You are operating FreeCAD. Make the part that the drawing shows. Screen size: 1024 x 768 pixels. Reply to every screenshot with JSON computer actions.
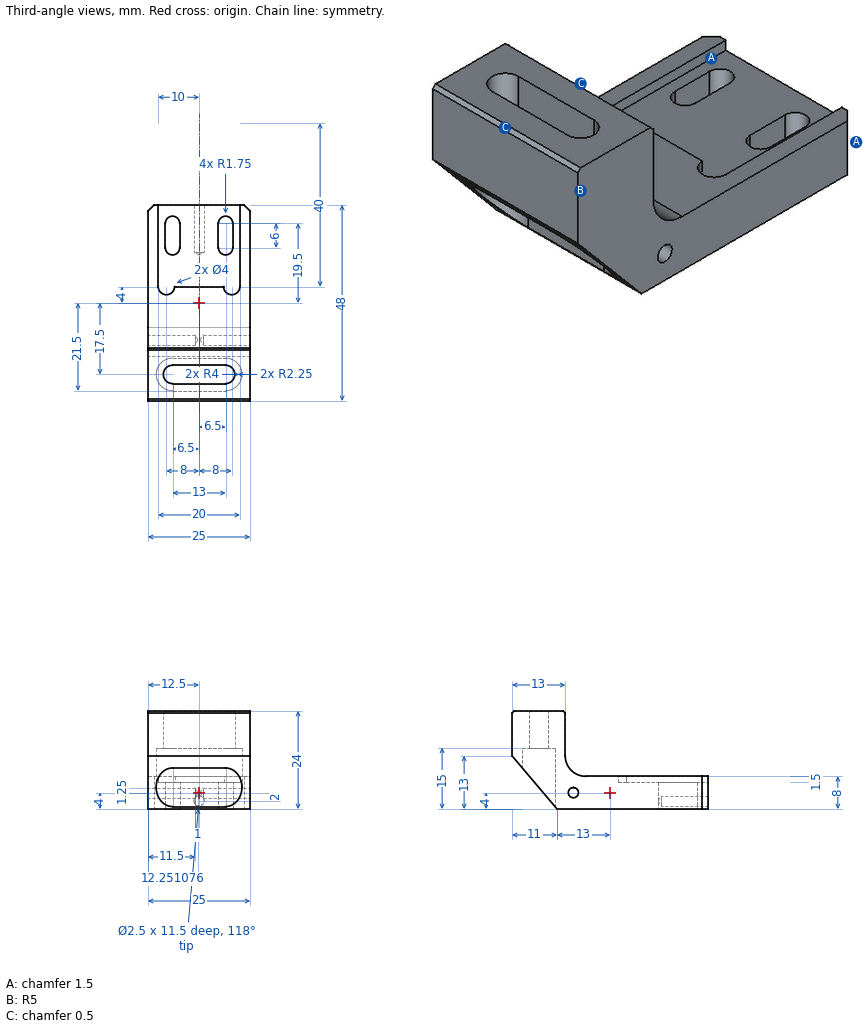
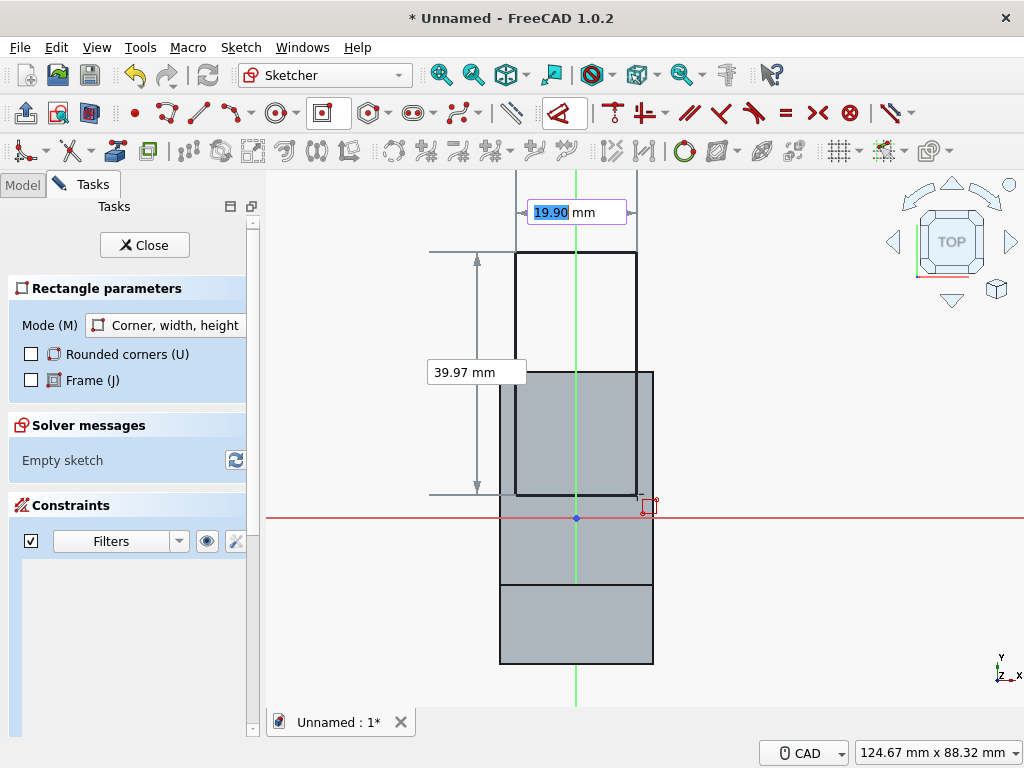
{"action": "type", "text": "20"}
{"action": "key", "text": "Tab"}
{"action": "type", "text": "40"}
{"action": "key", "text": "Return"}
{"action": "key", "text": "Escape"}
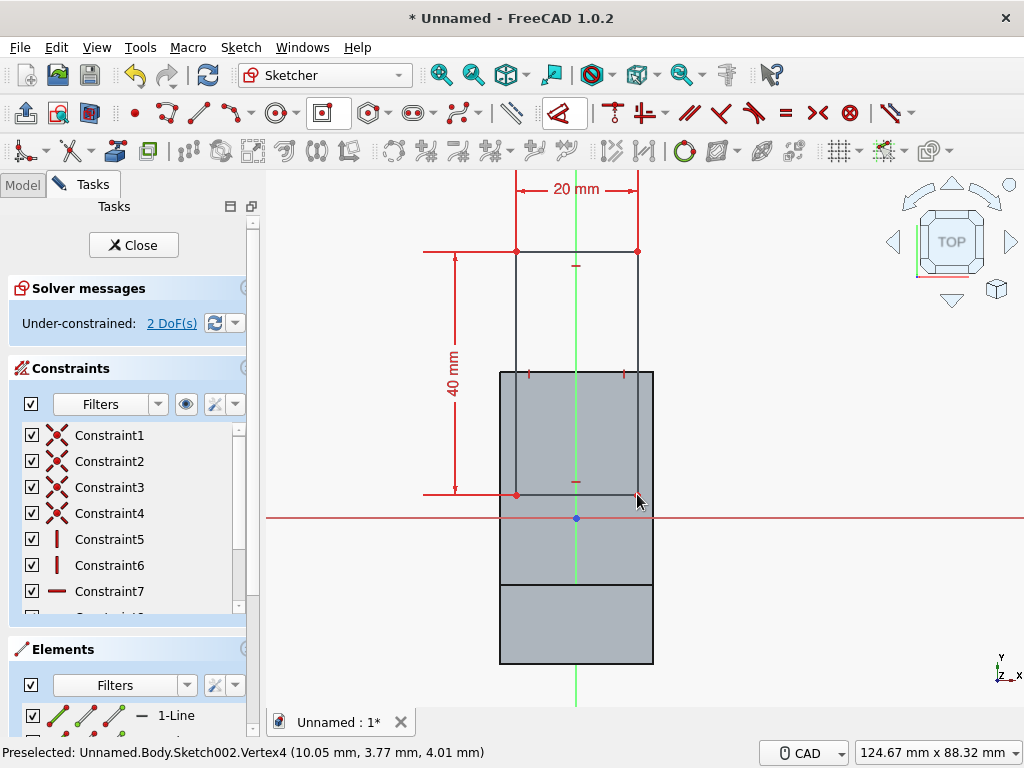
{"action": "scroll", "coordinate": [516, 495], "scroll_direction": "up", "scroll_amount": 3}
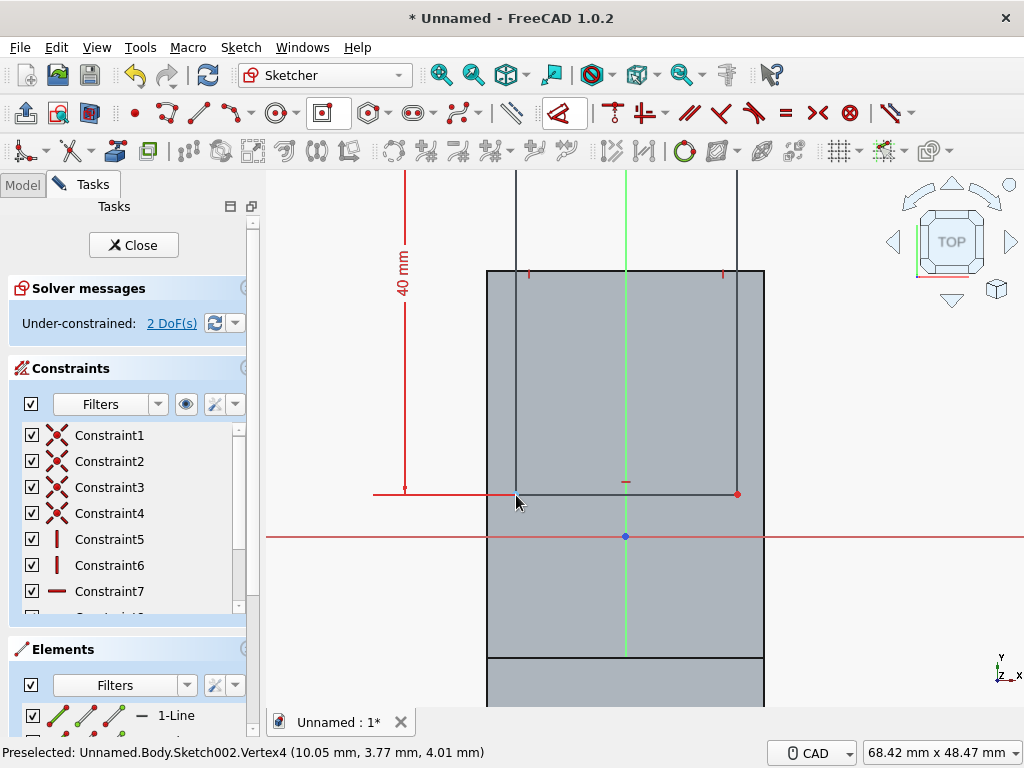
{"action": "left_click", "coordinate": [516, 495]}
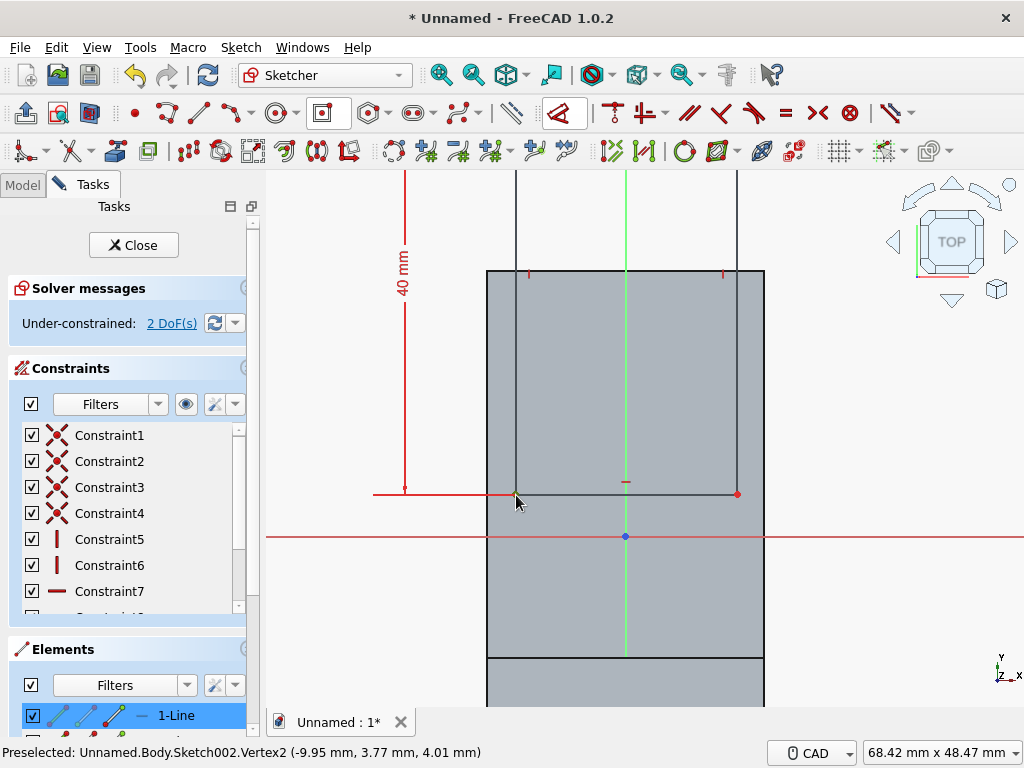
{"action": "left_click", "coordinate": [582, 114]}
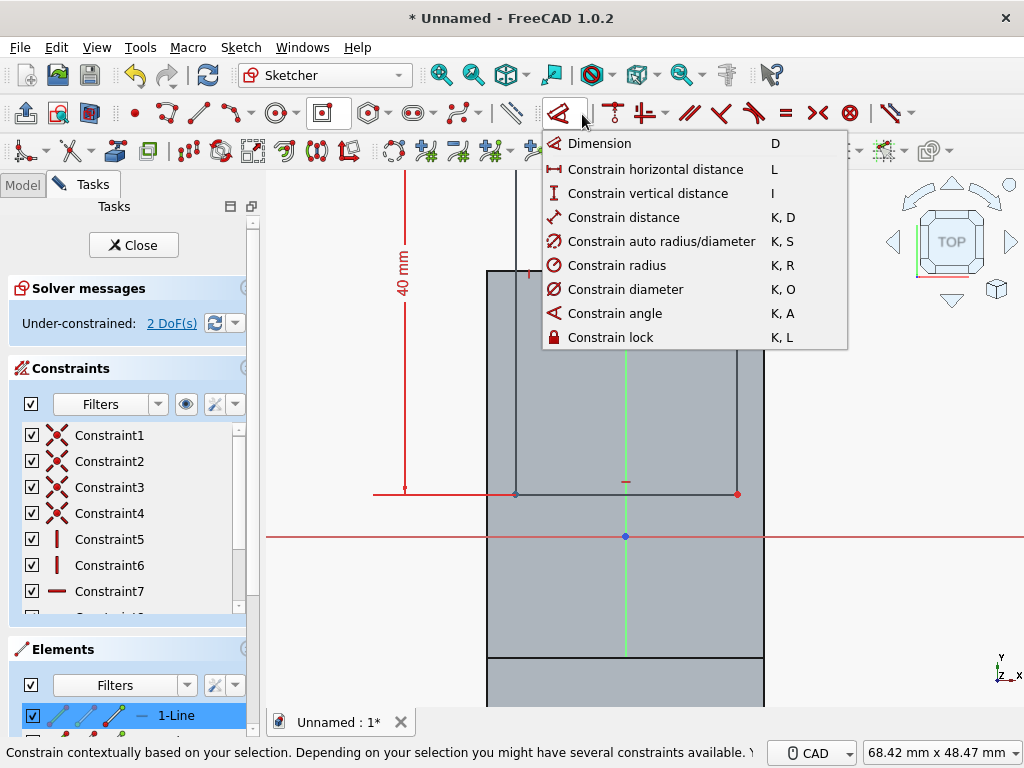
{"action": "left_click", "coordinate": [695, 193]}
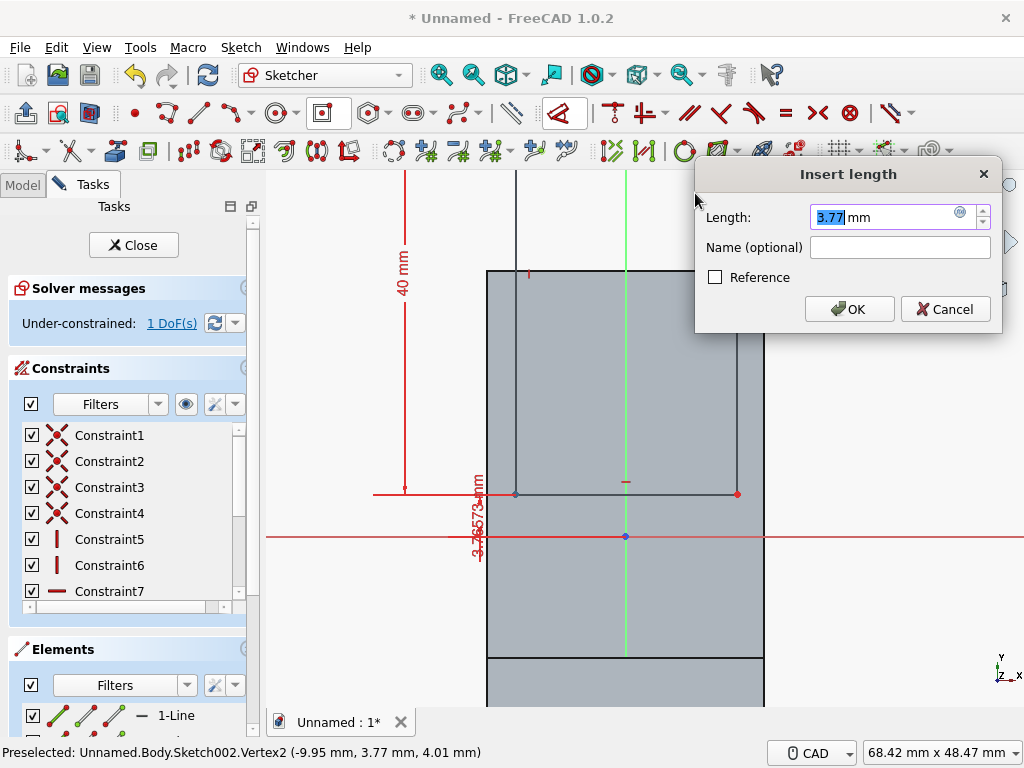
{"action": "type", "text": "4"}
{"action": "key", "text": "Return"}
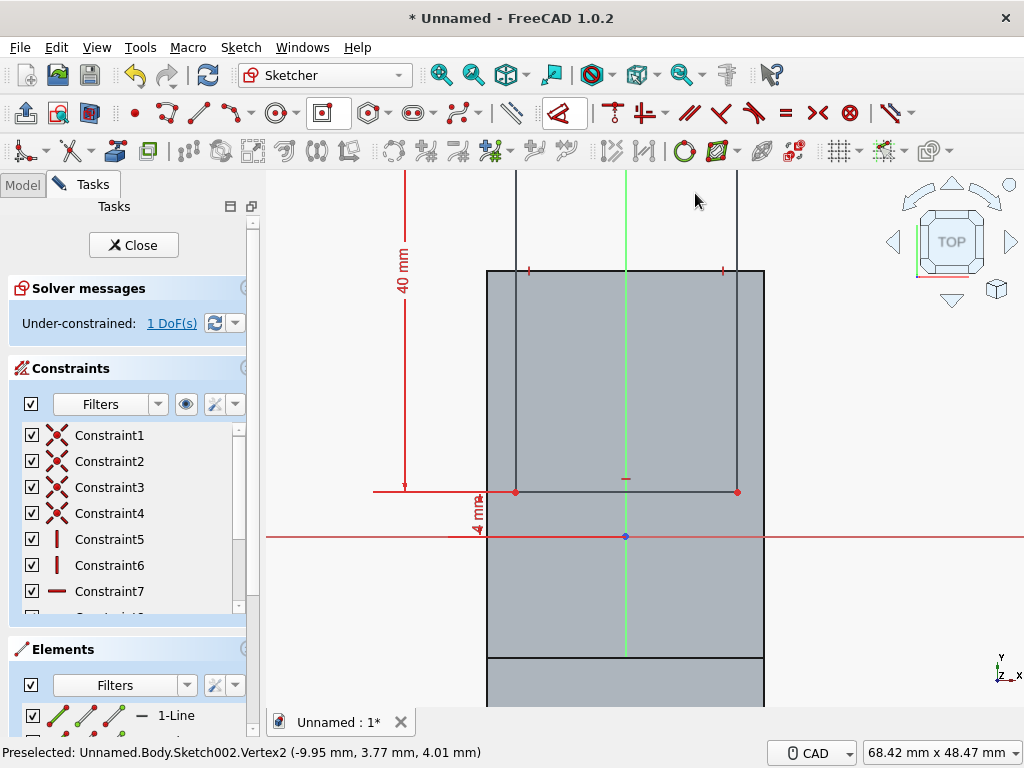
{"action": "scroll", "coordinate": [476, 679], "scroll_direction": "down", "scroll_amount": 2}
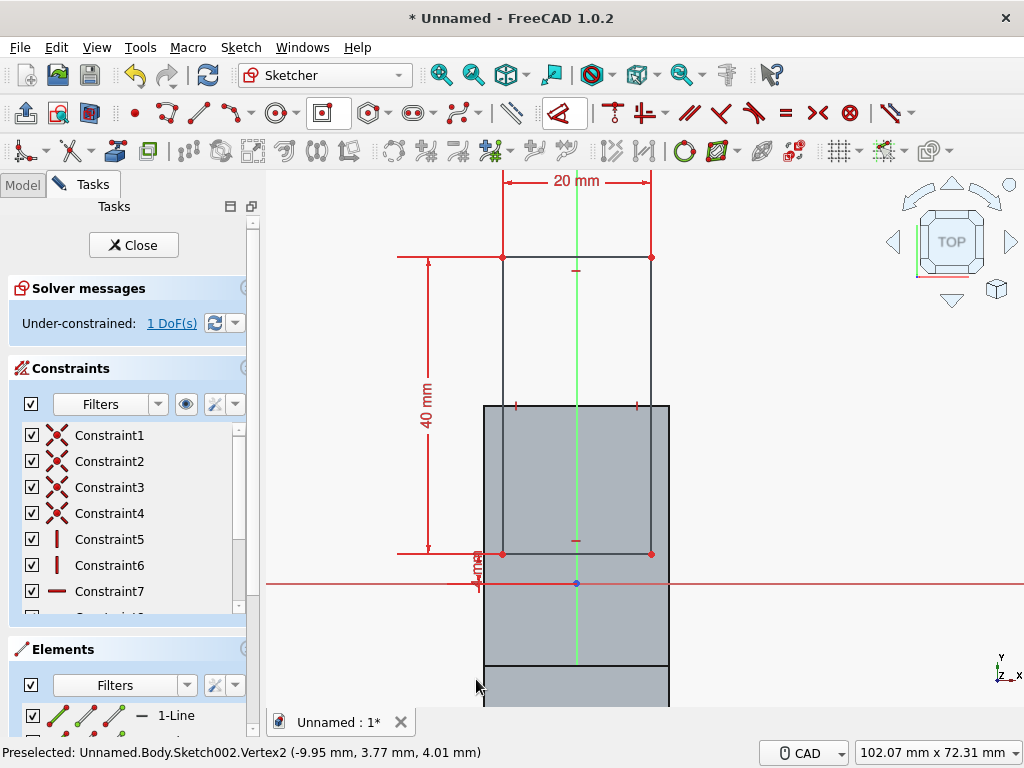
{"action": "left_click", "coordinate": [503, 257]}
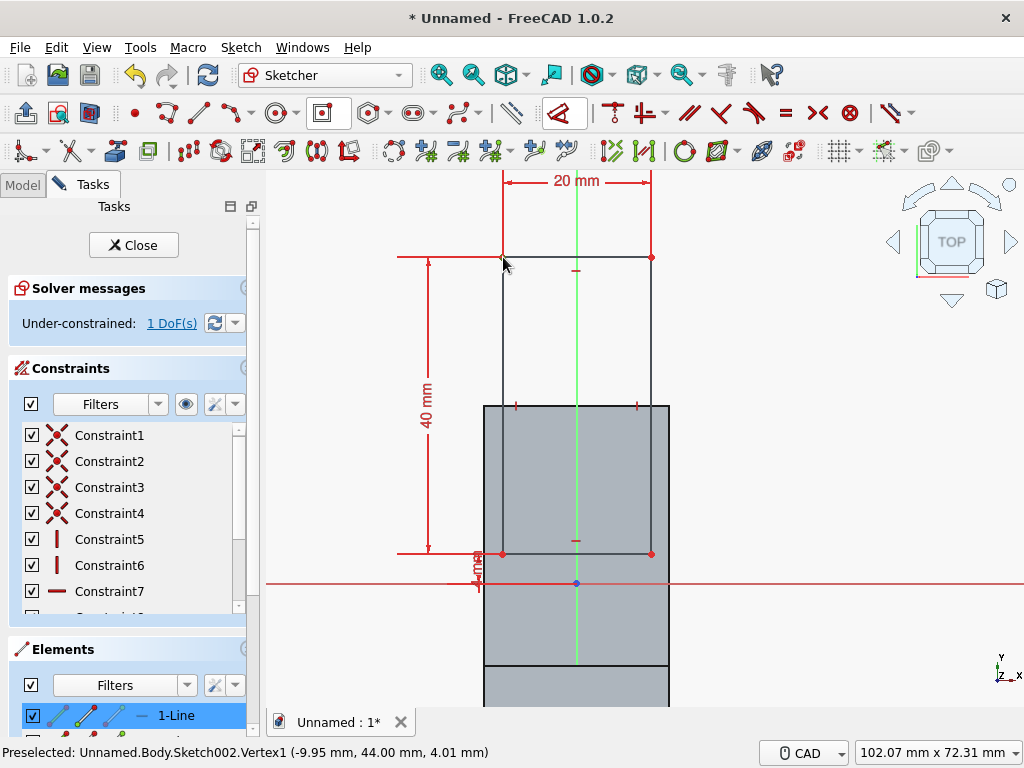
{"action": "left_click", "coordinate": [582, 114]}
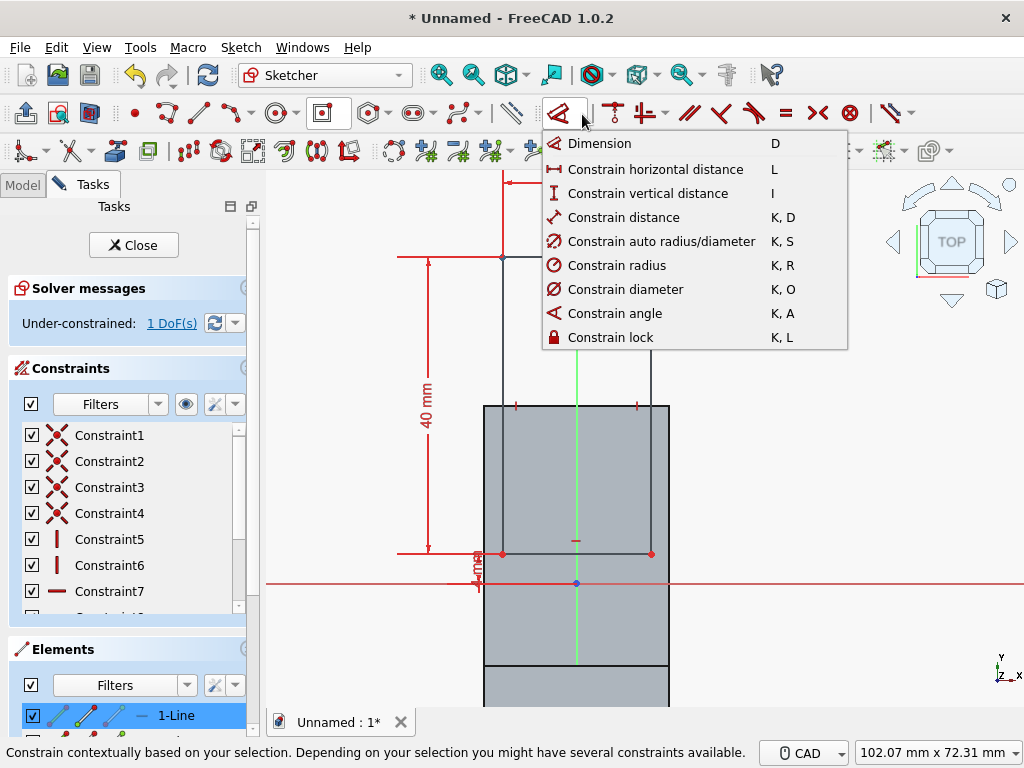
{"action": "left_click", "coordinate": [695, 169]}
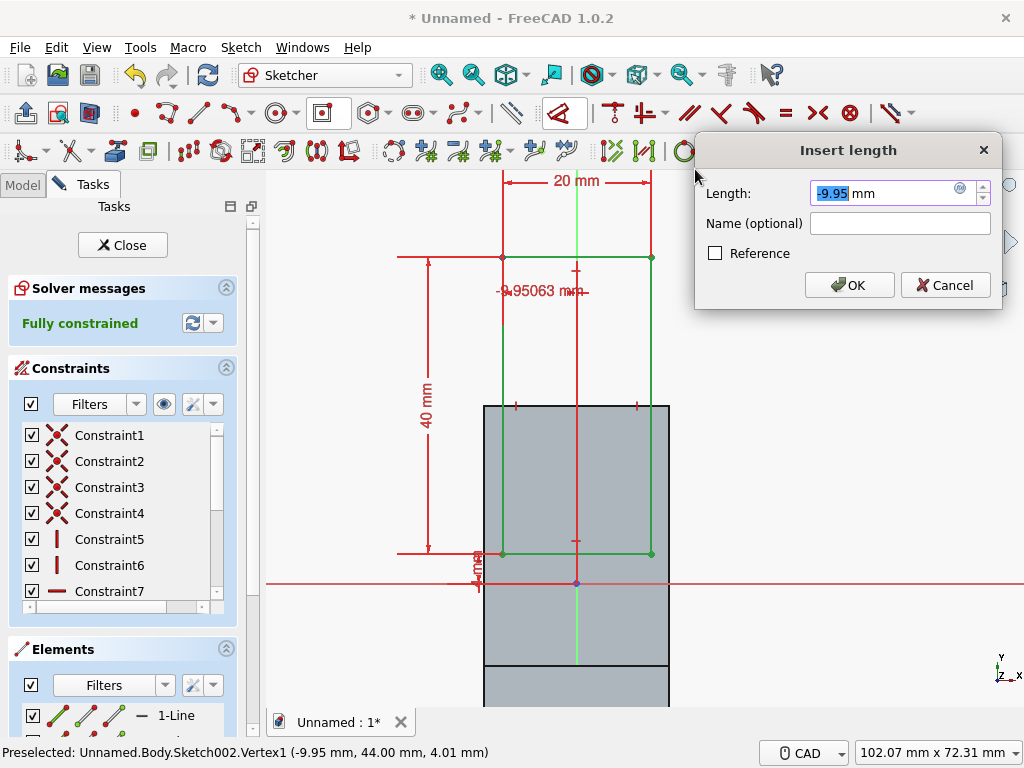
{"action": "type", "text": "-10"}
{"action": "key", "text": "Return"}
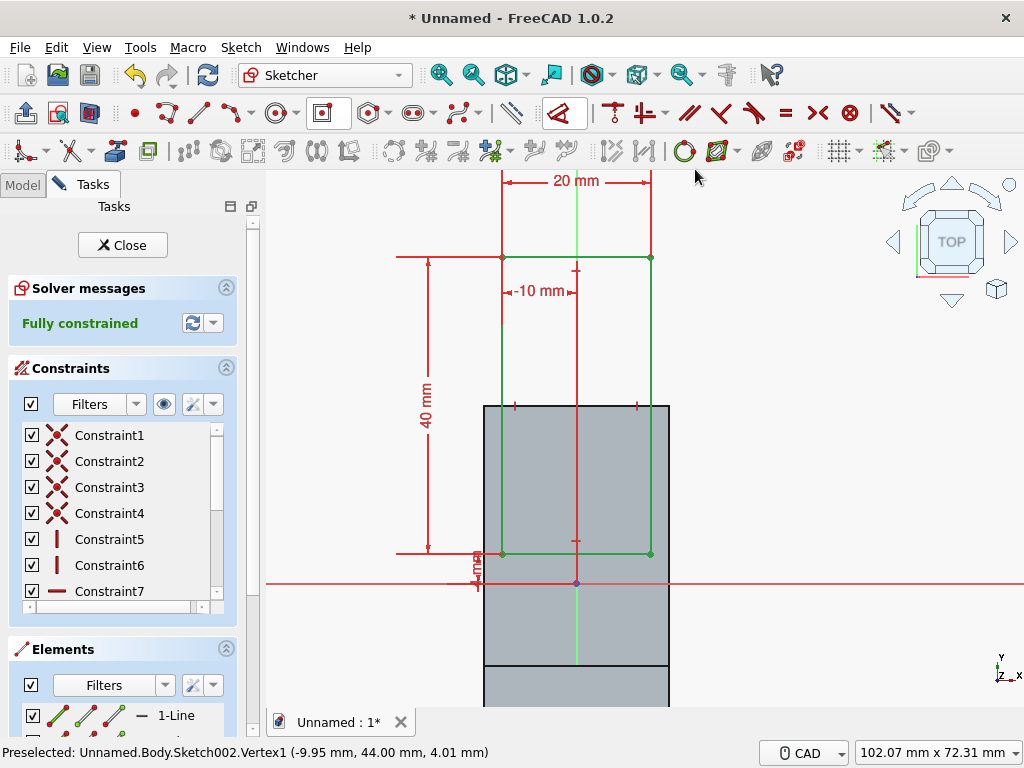
{"action": "left_click", "coordinate": [123, 245]}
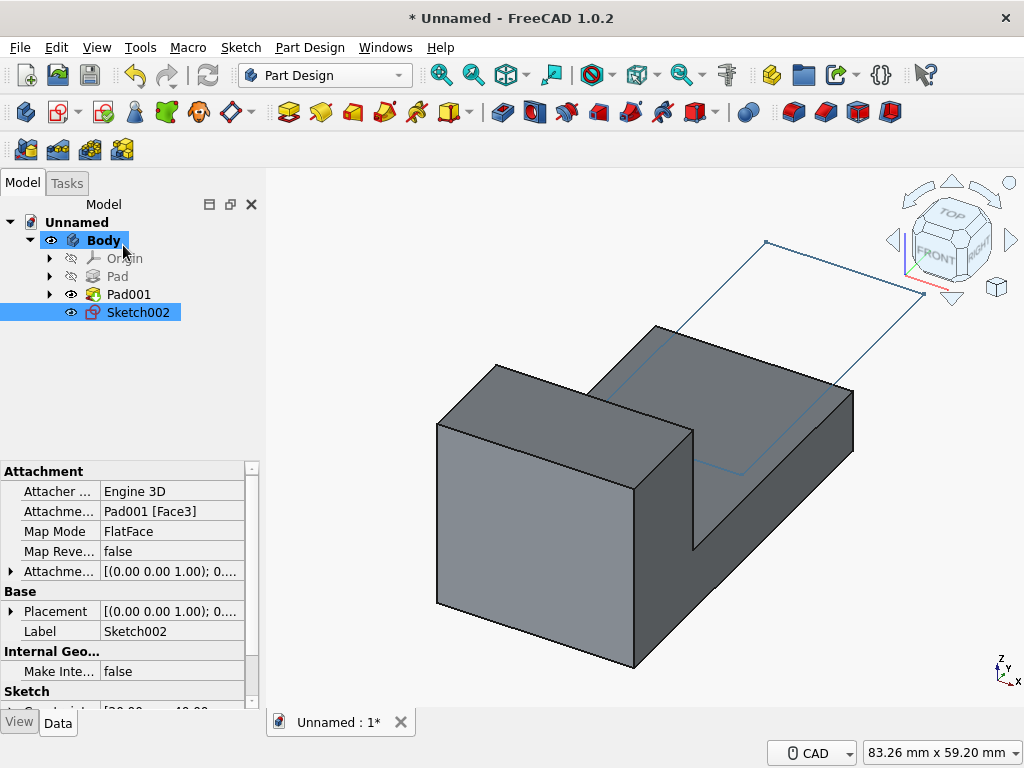
{"action": "left_click", "coordinate": [504, 112]}